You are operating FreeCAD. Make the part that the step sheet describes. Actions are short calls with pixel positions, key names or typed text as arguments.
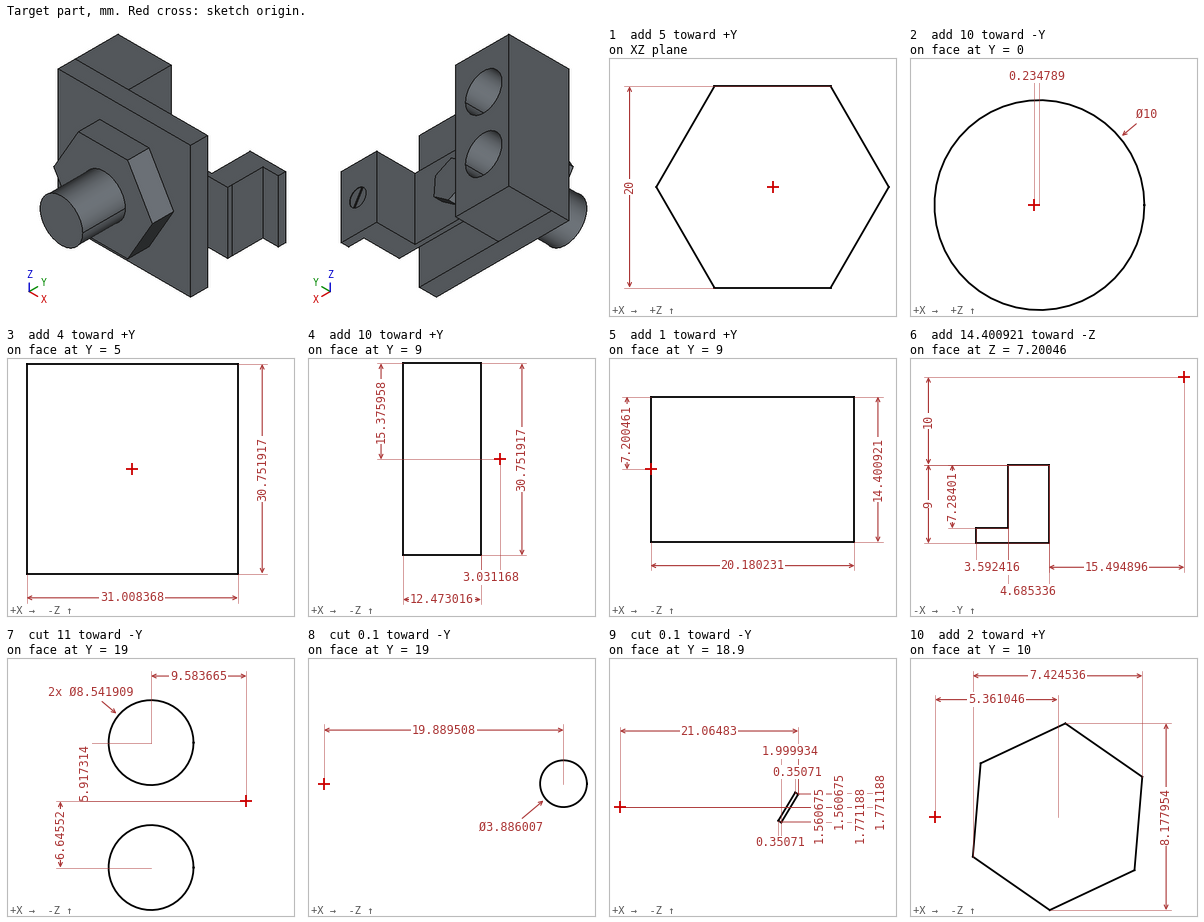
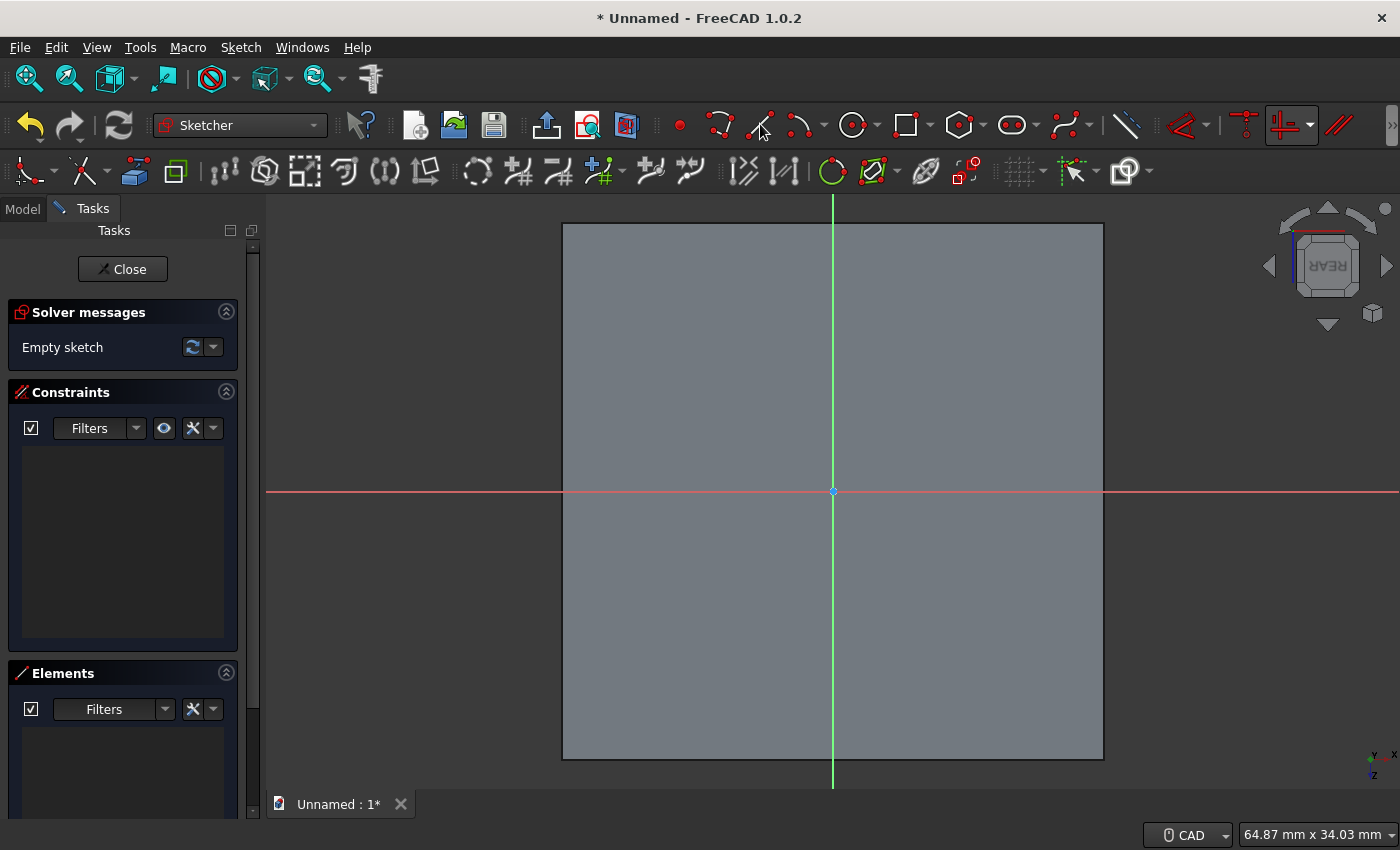
scroll(901, 492, down, 2)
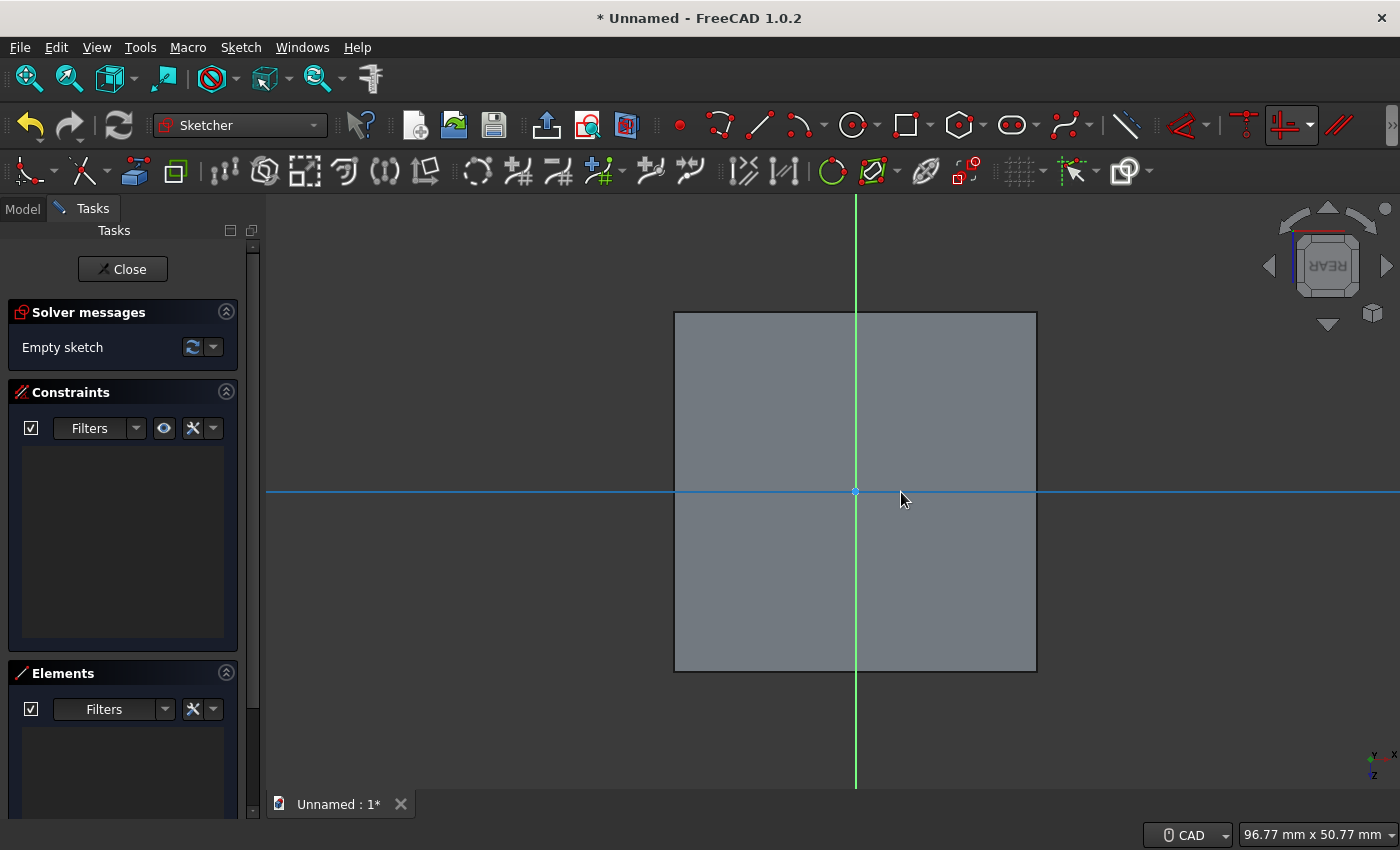
click(906, 126)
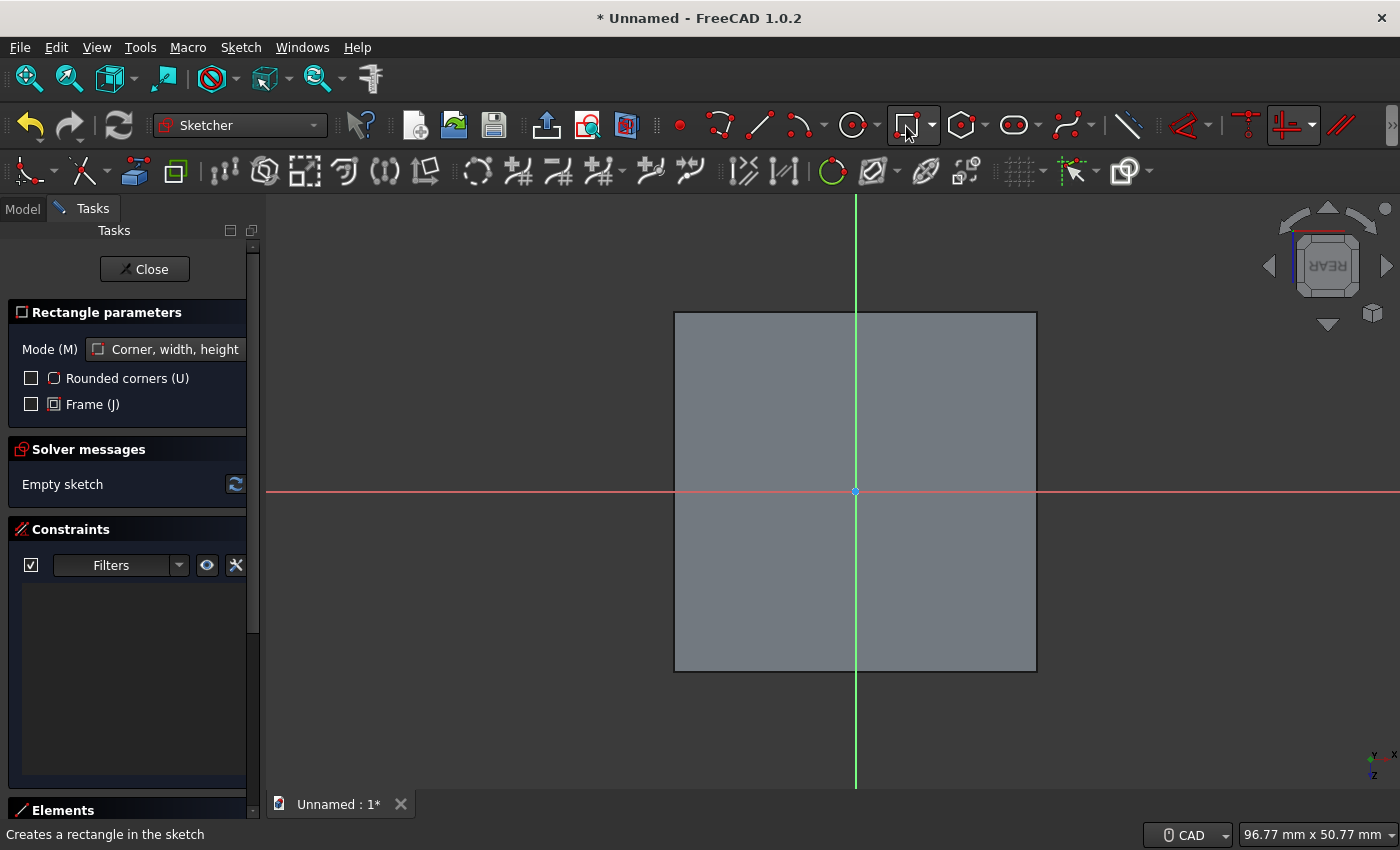
click(674, 312)
move(820, 672)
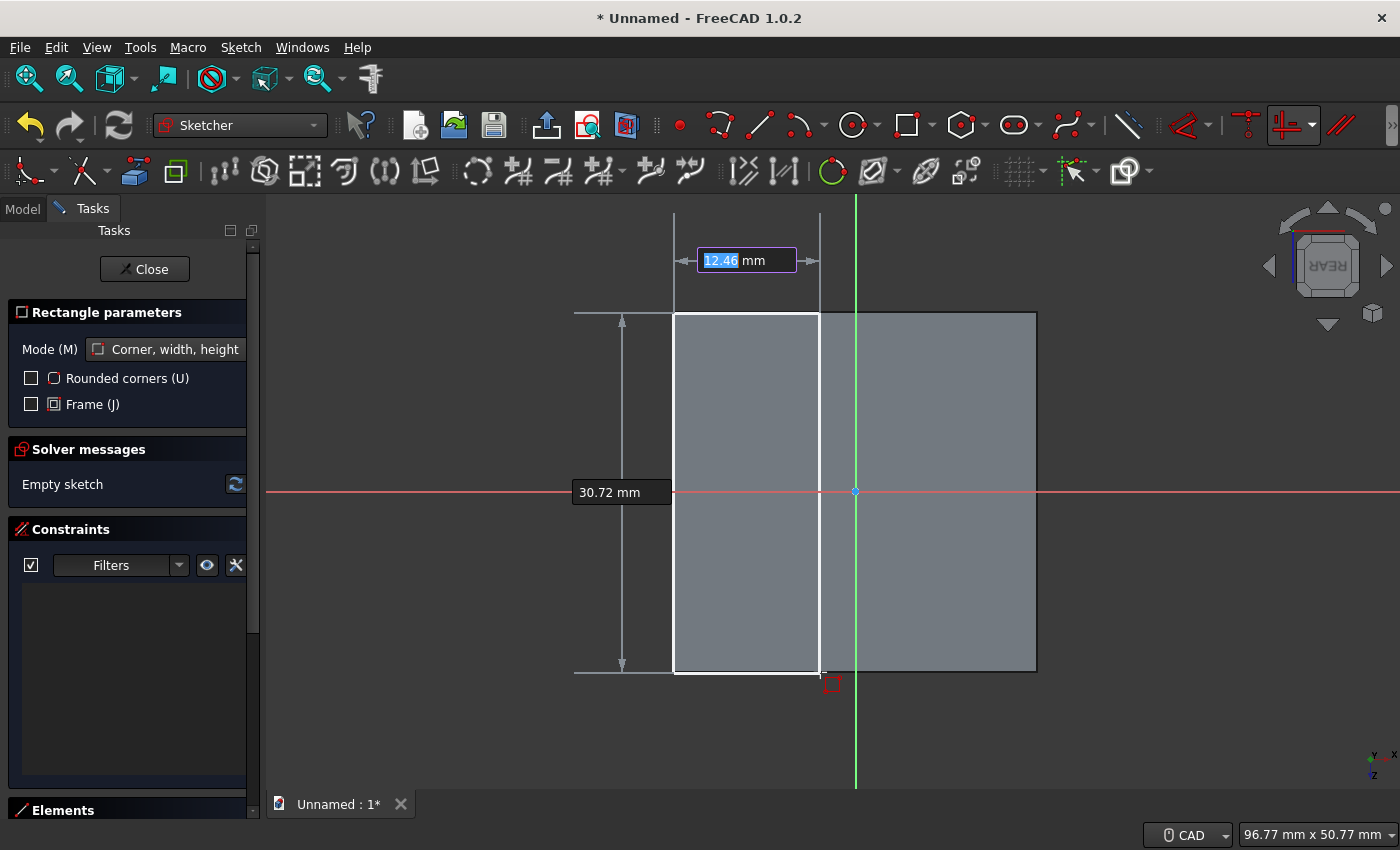
text(12.473016)
key(Tab)
text(30.751917)
key(Return)
key(Escape)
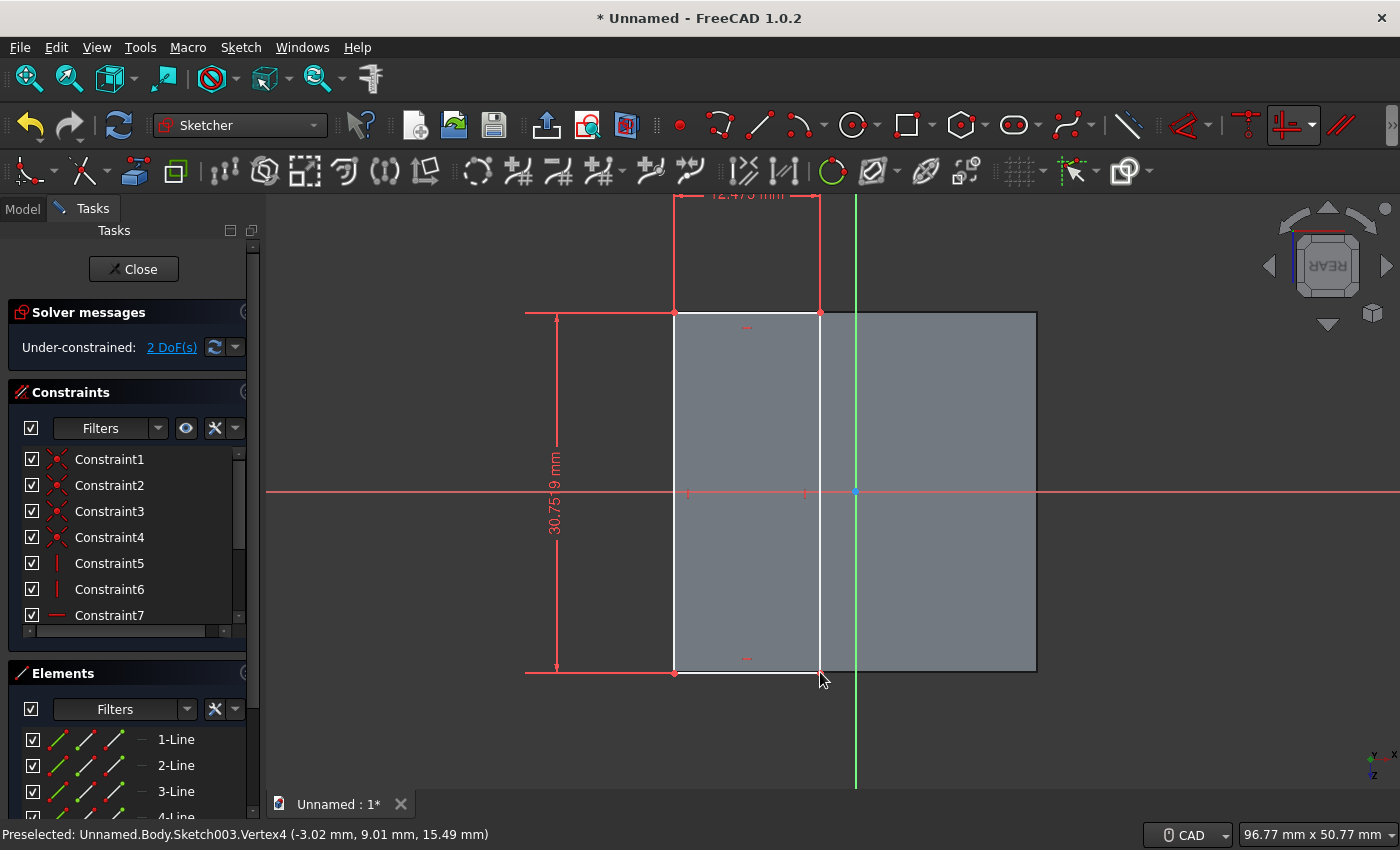
click(1184, 126)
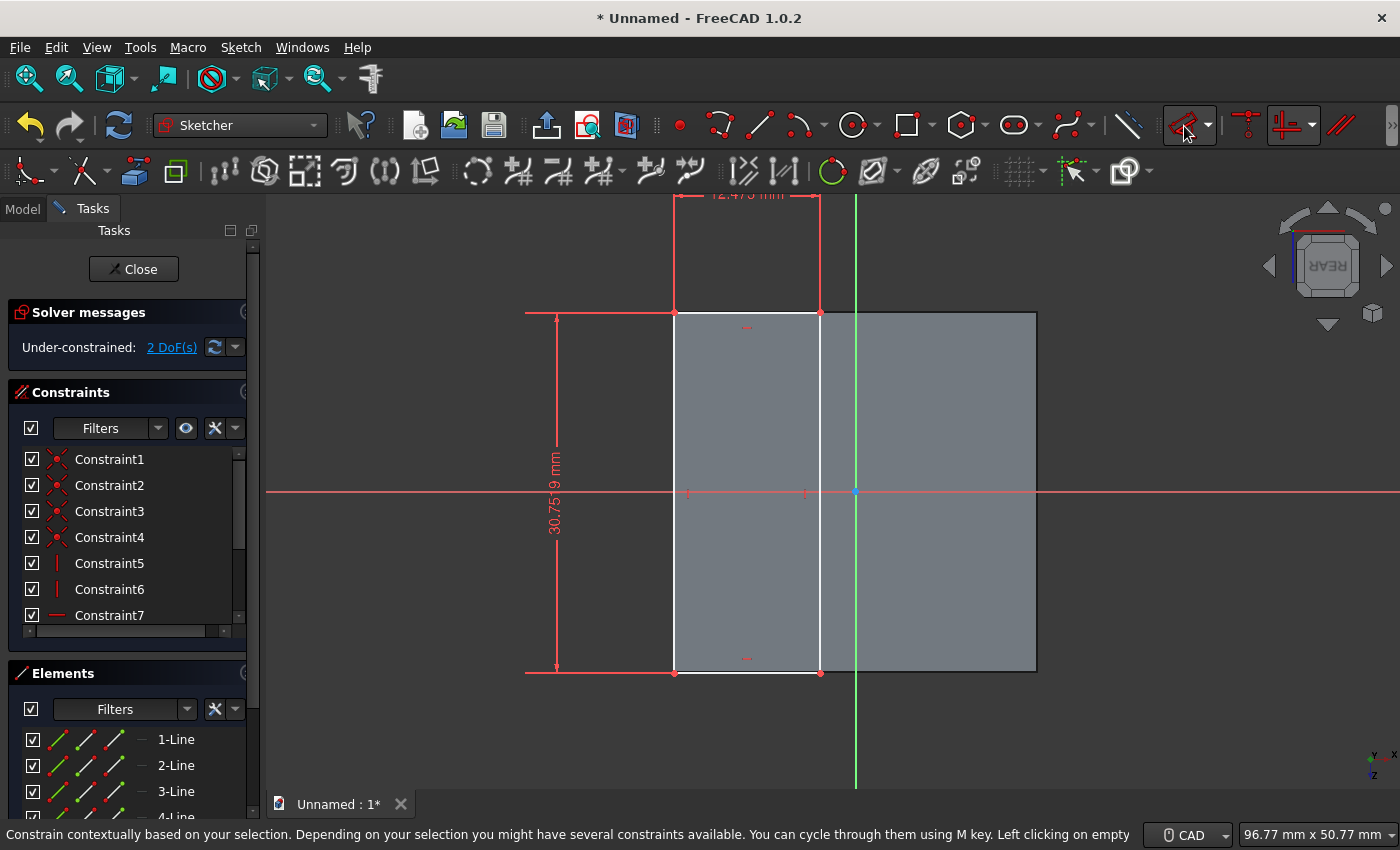
click(820, 673)
click(838, 707)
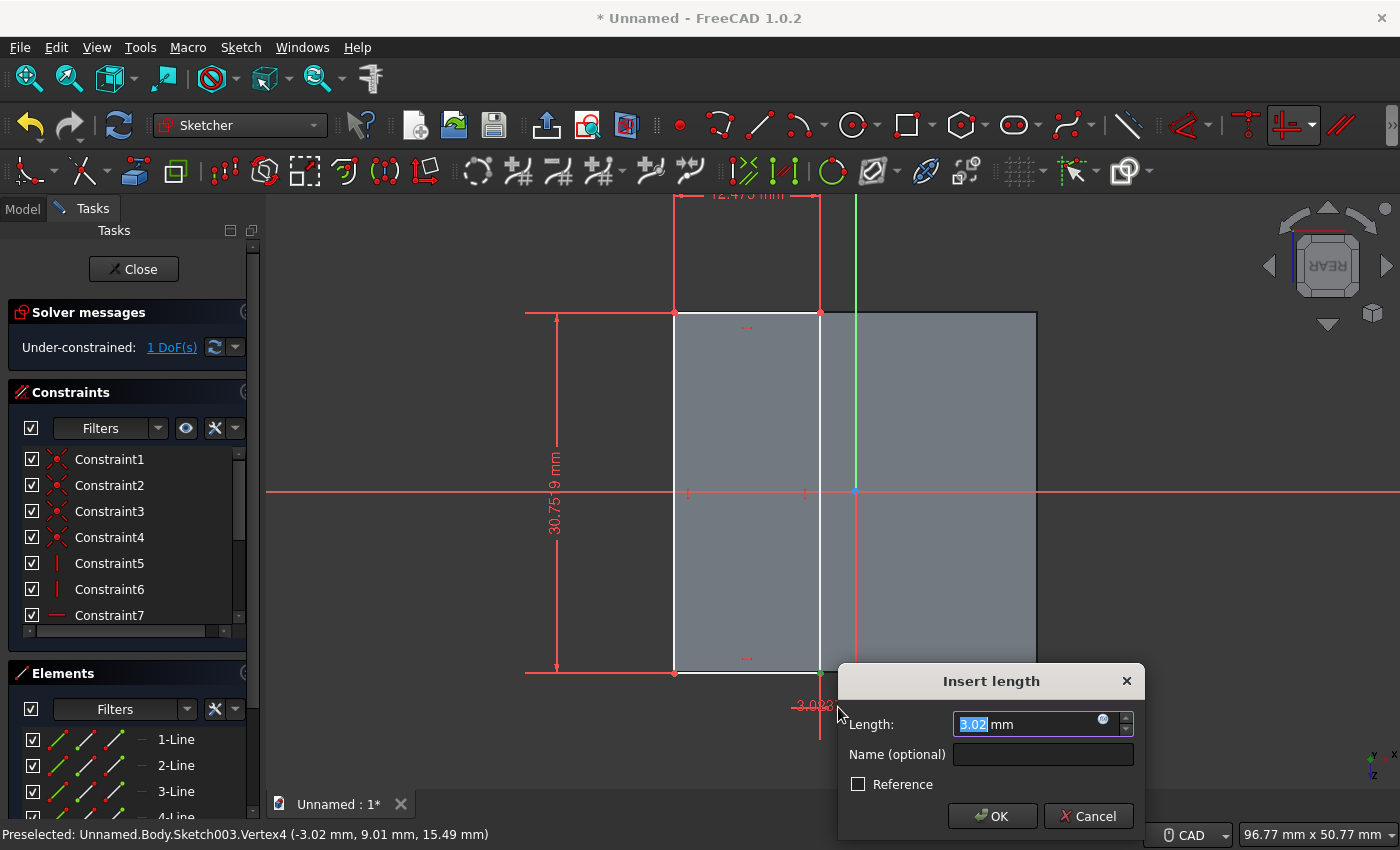
text(3.031168)
key(Return)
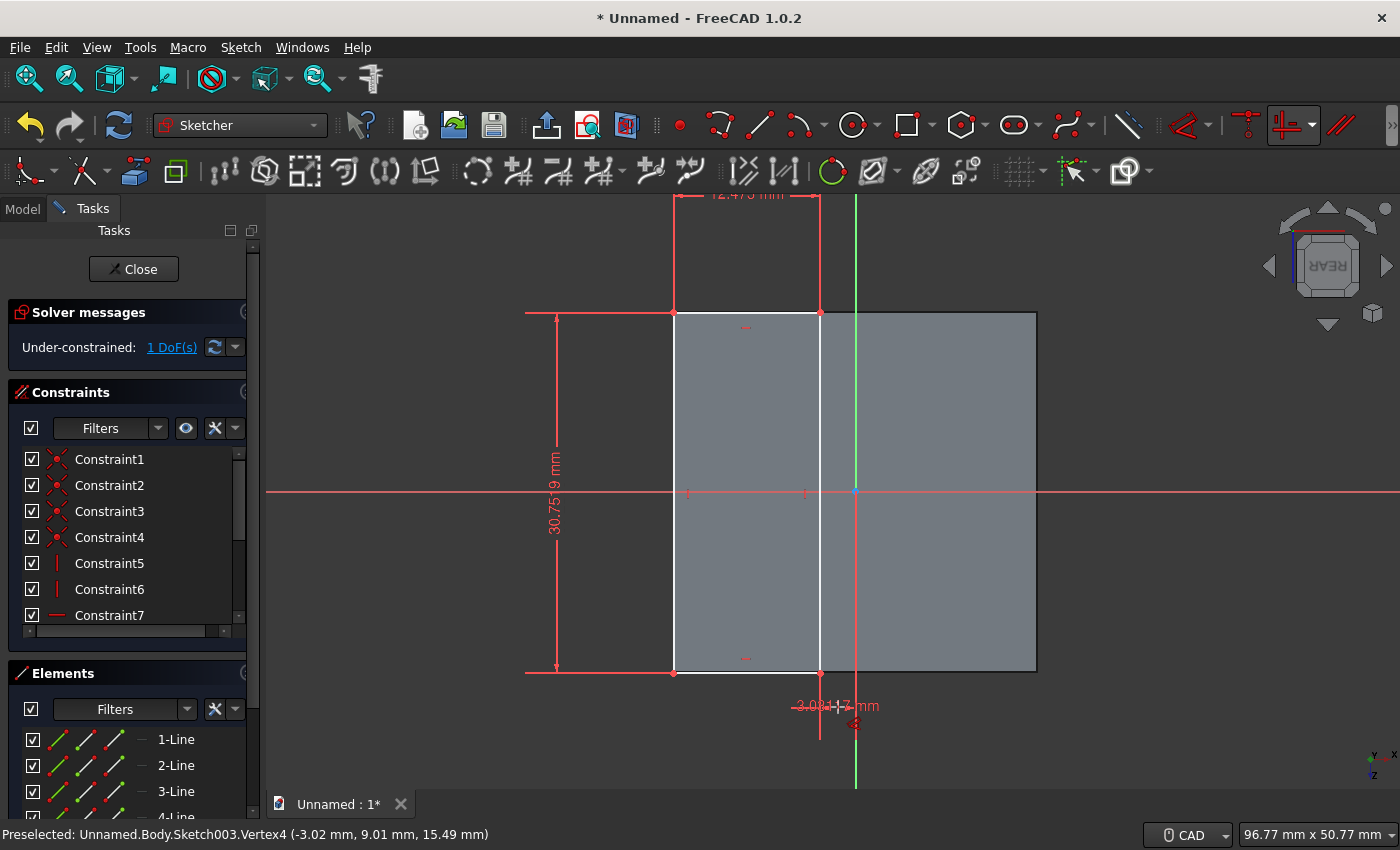
click(674, 313)
click(890, 402)